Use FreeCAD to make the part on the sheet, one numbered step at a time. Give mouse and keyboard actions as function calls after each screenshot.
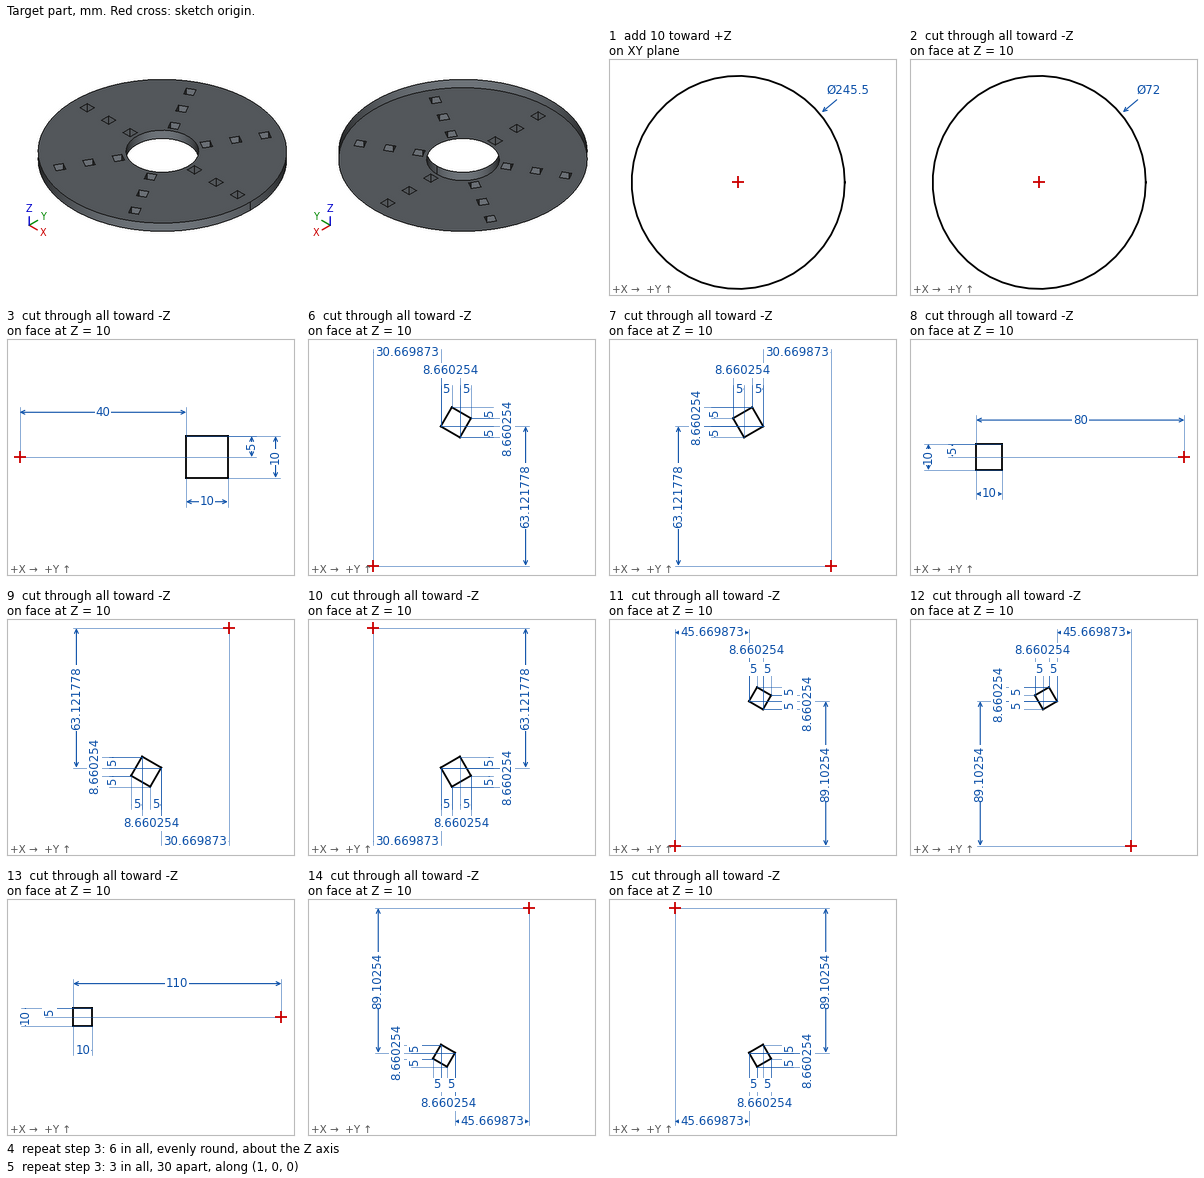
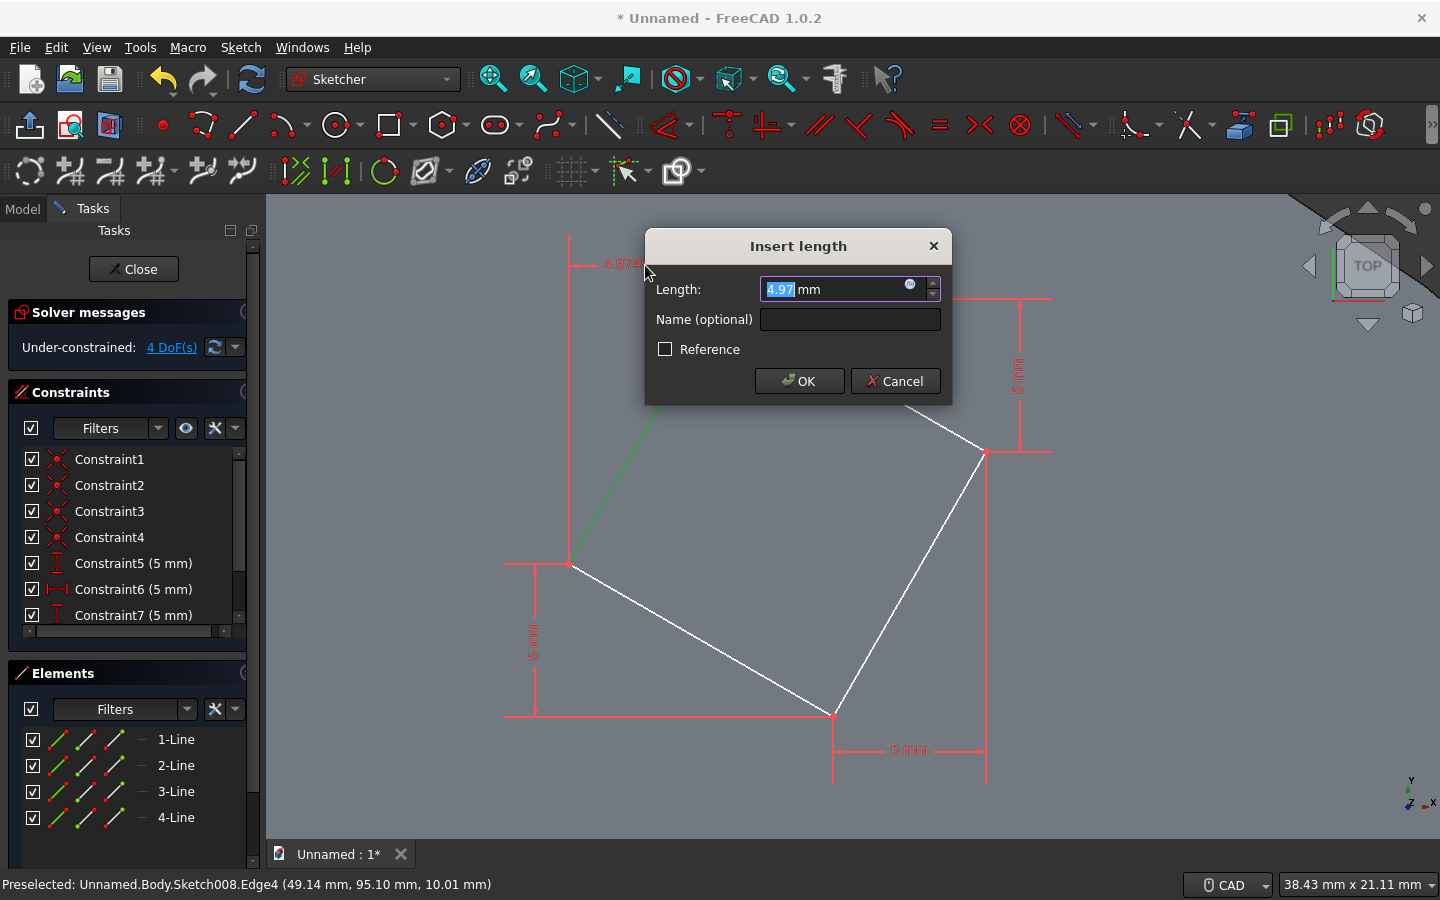
text(5)
key(Return)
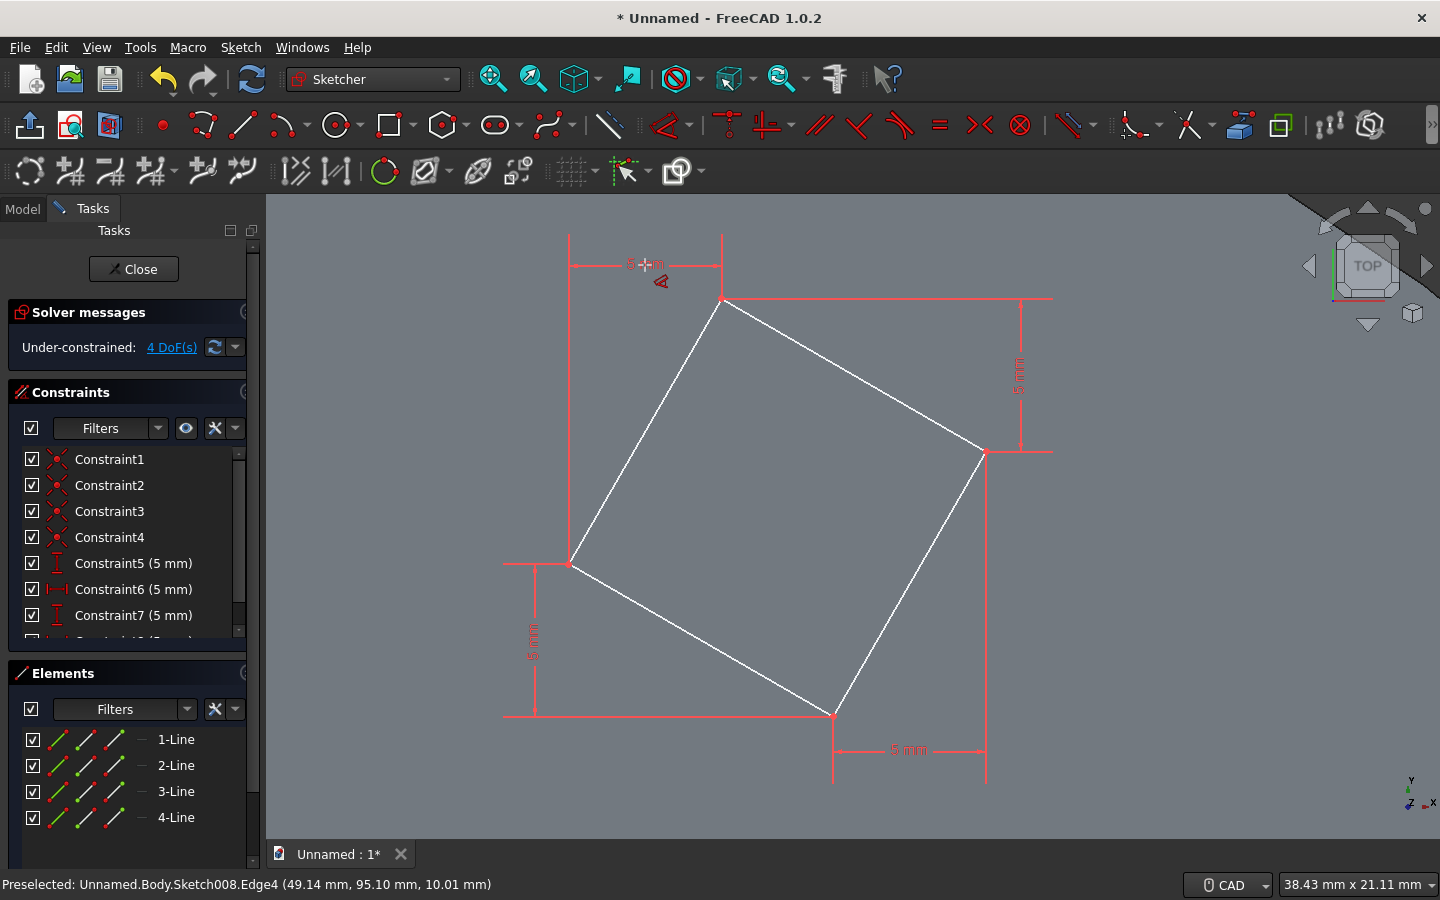
click(569, 564)
click(603, 688)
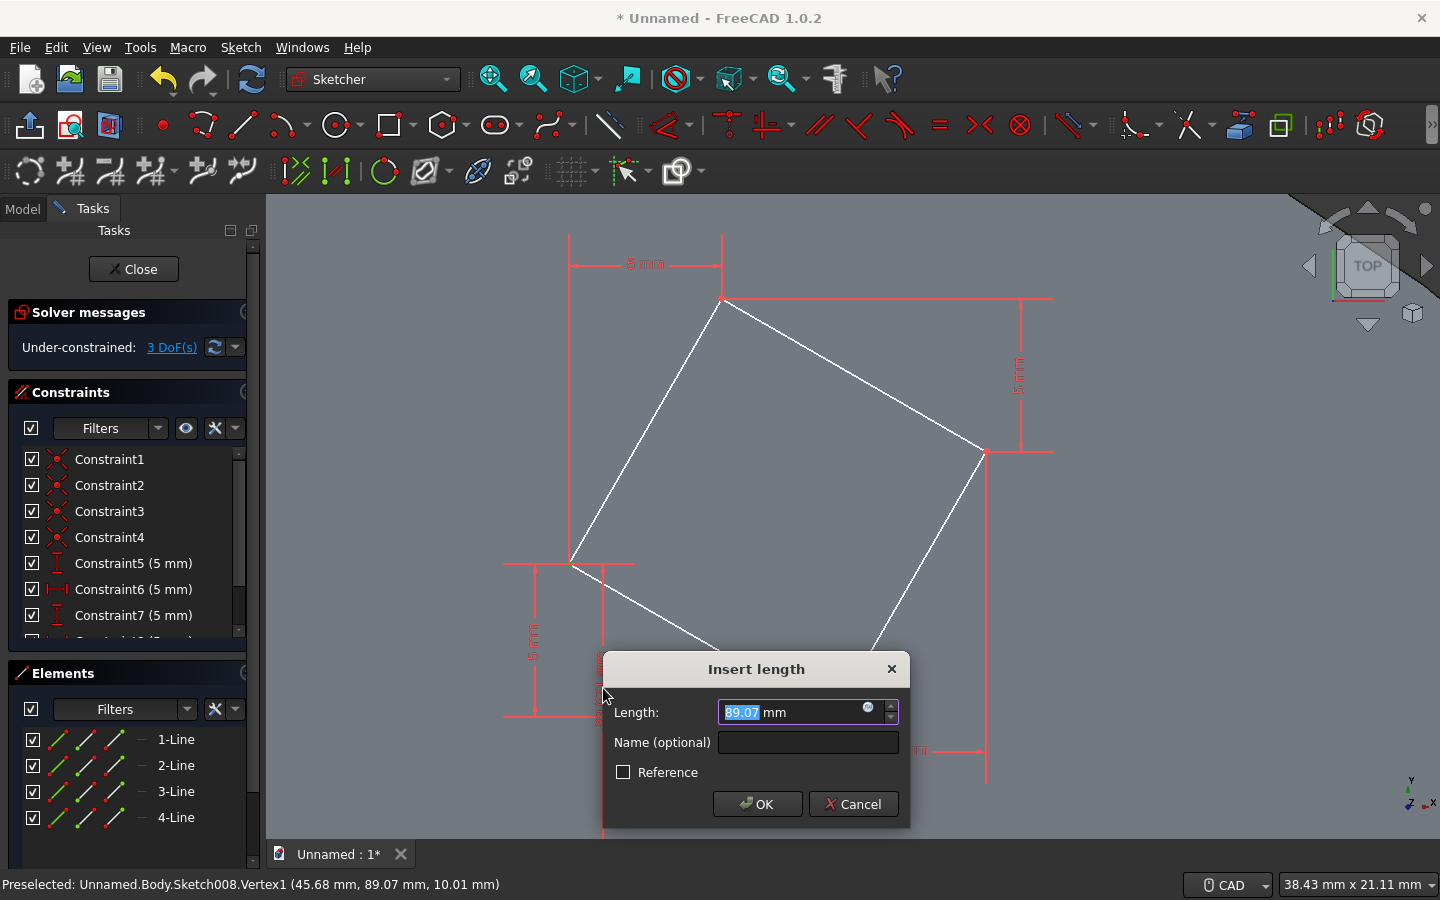
text(89.10254)
key(Return)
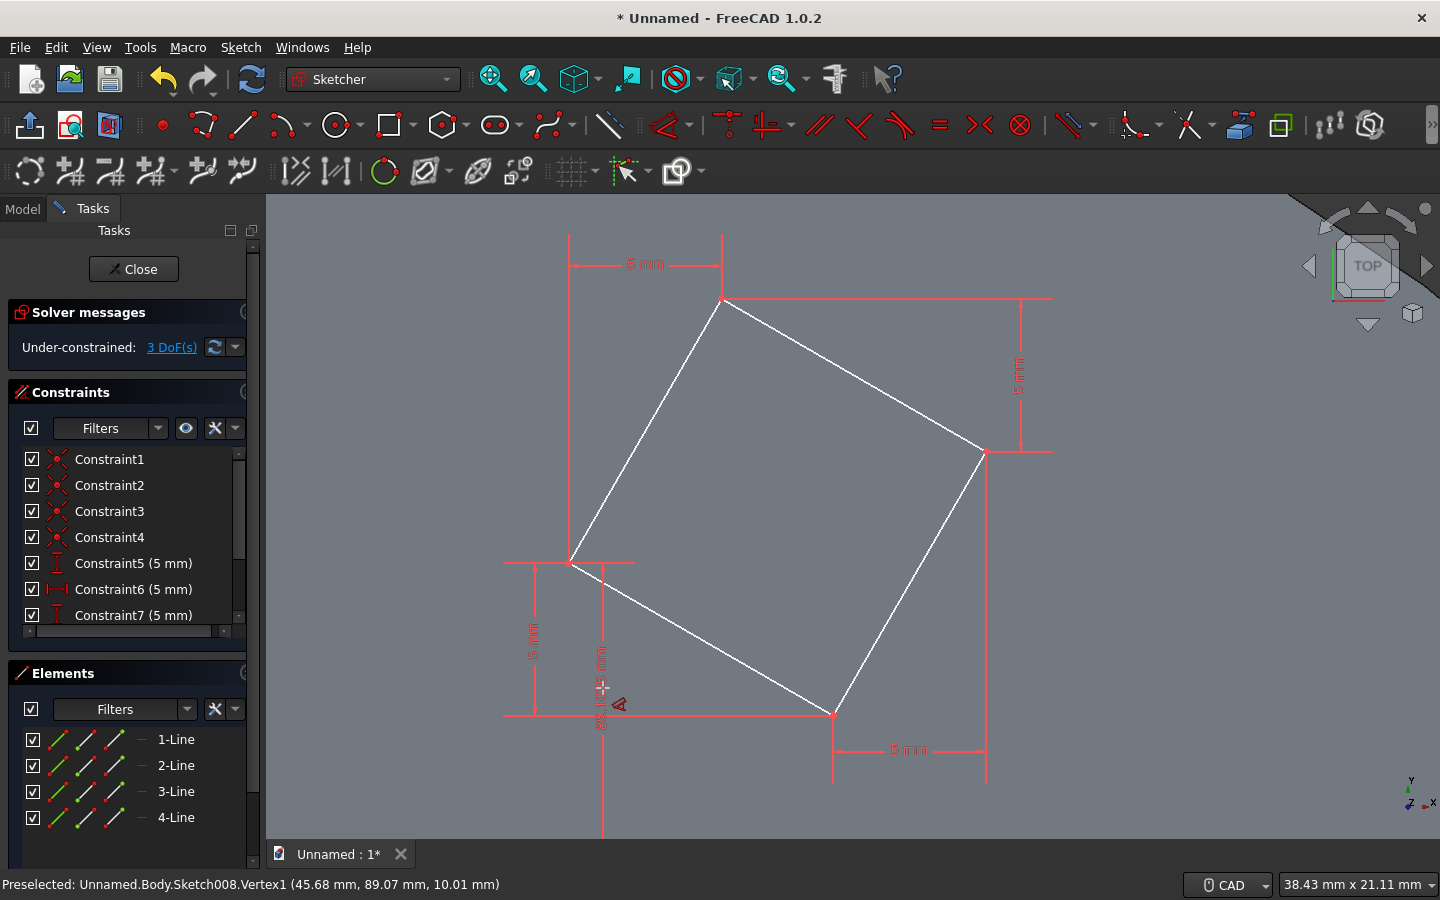
click(648, 609)
click(701, 750)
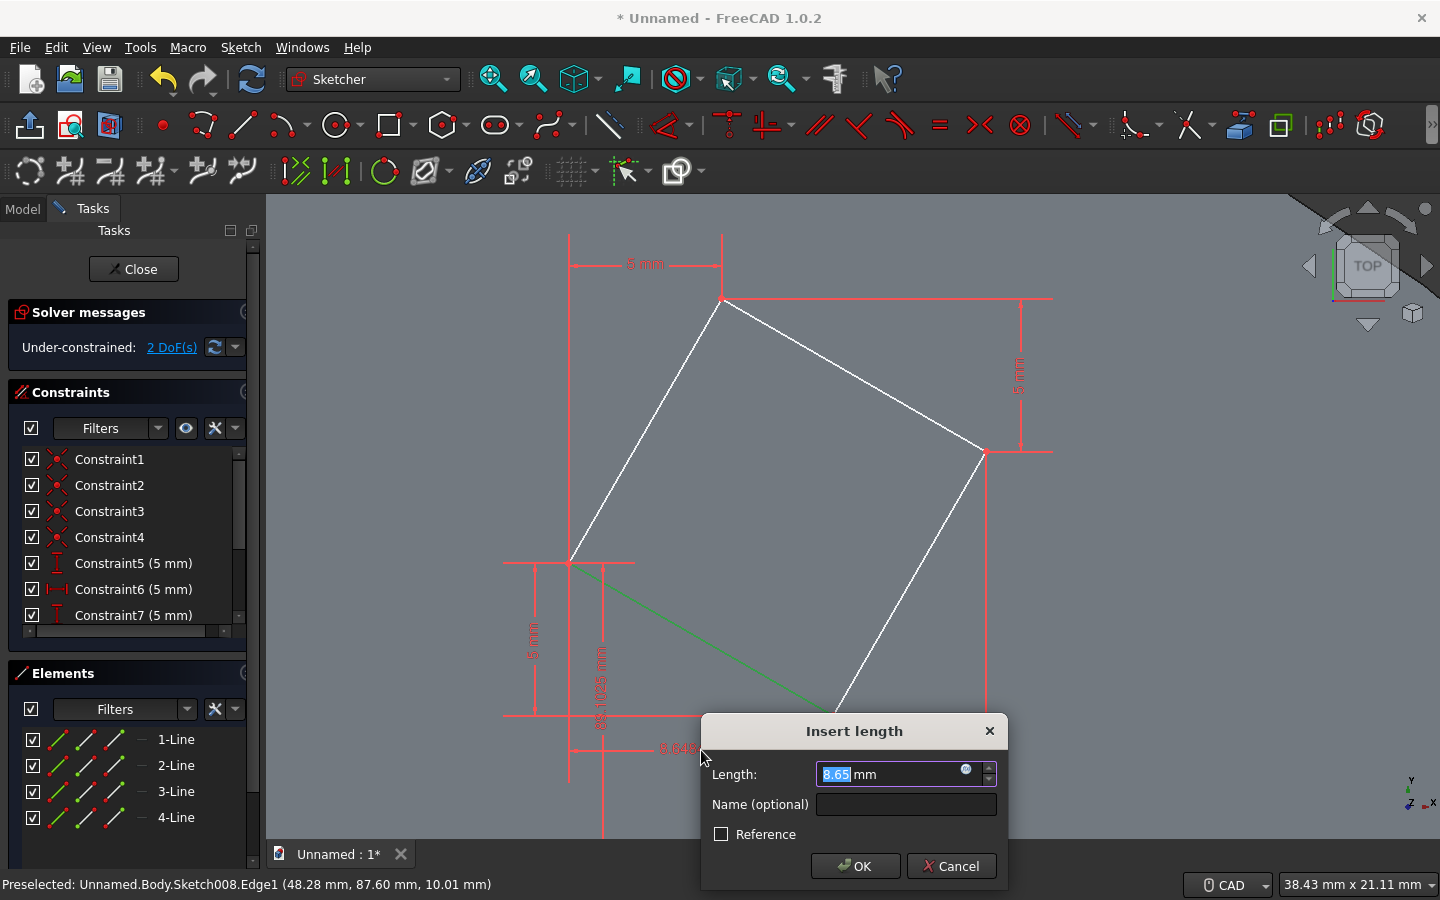
text(8.660254)
key(Return)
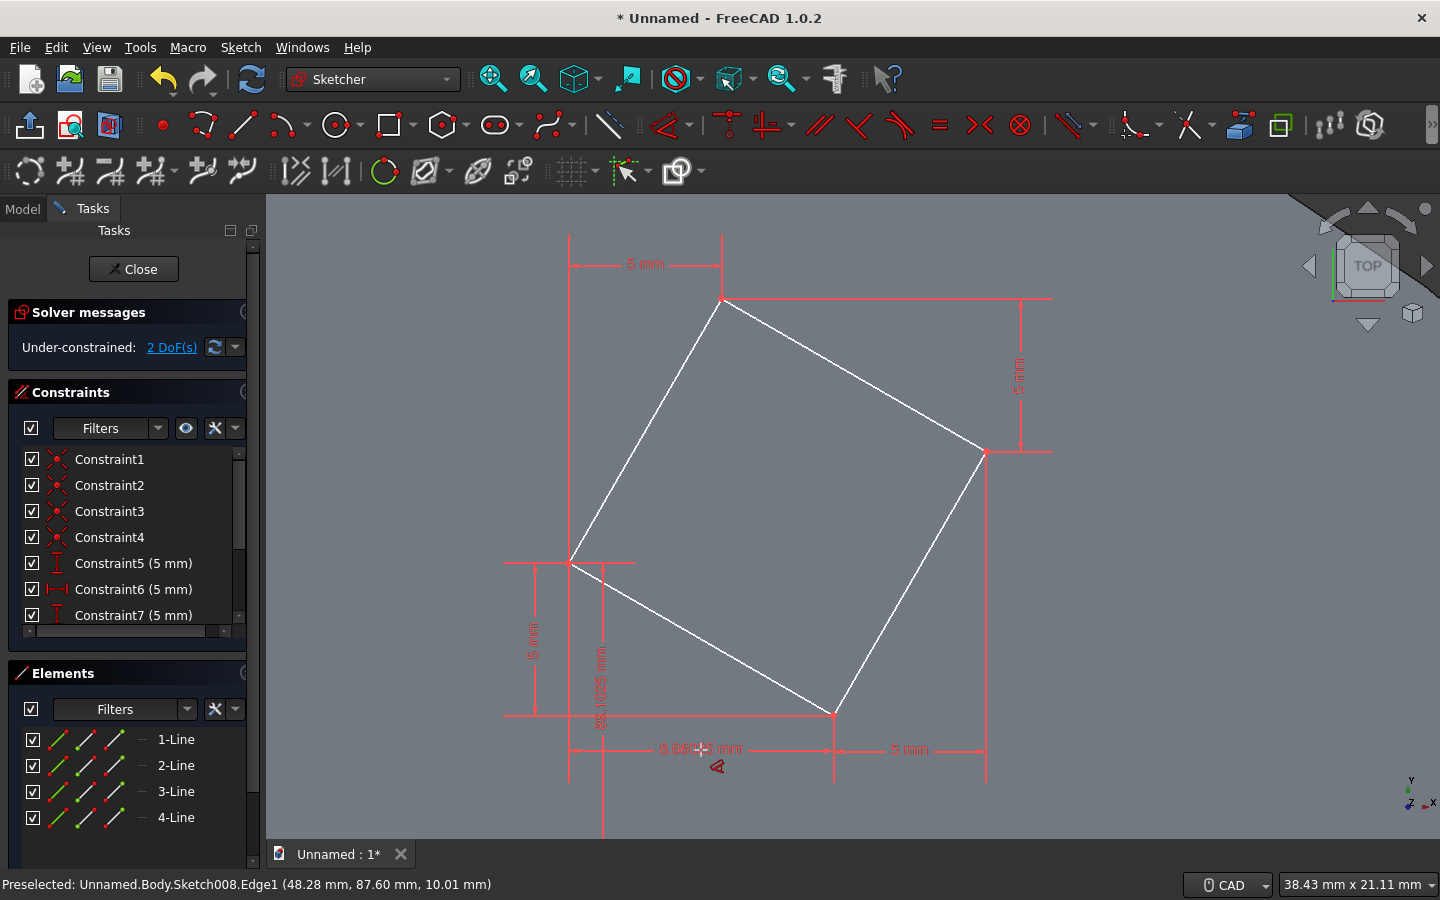
click(879, 637)
click(1020, 584)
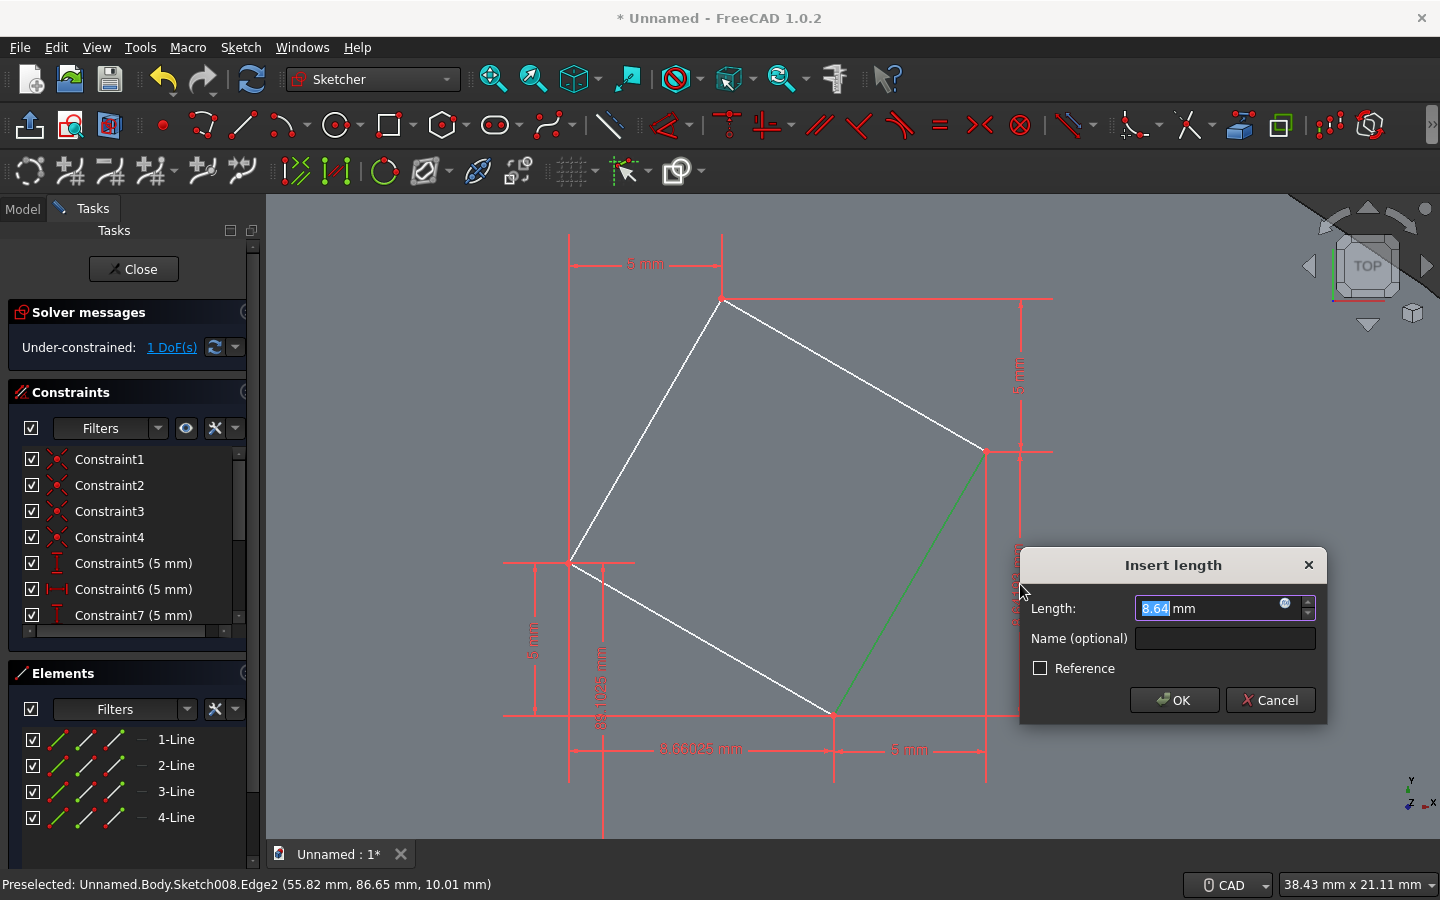
text(8.660254)
key(Return)